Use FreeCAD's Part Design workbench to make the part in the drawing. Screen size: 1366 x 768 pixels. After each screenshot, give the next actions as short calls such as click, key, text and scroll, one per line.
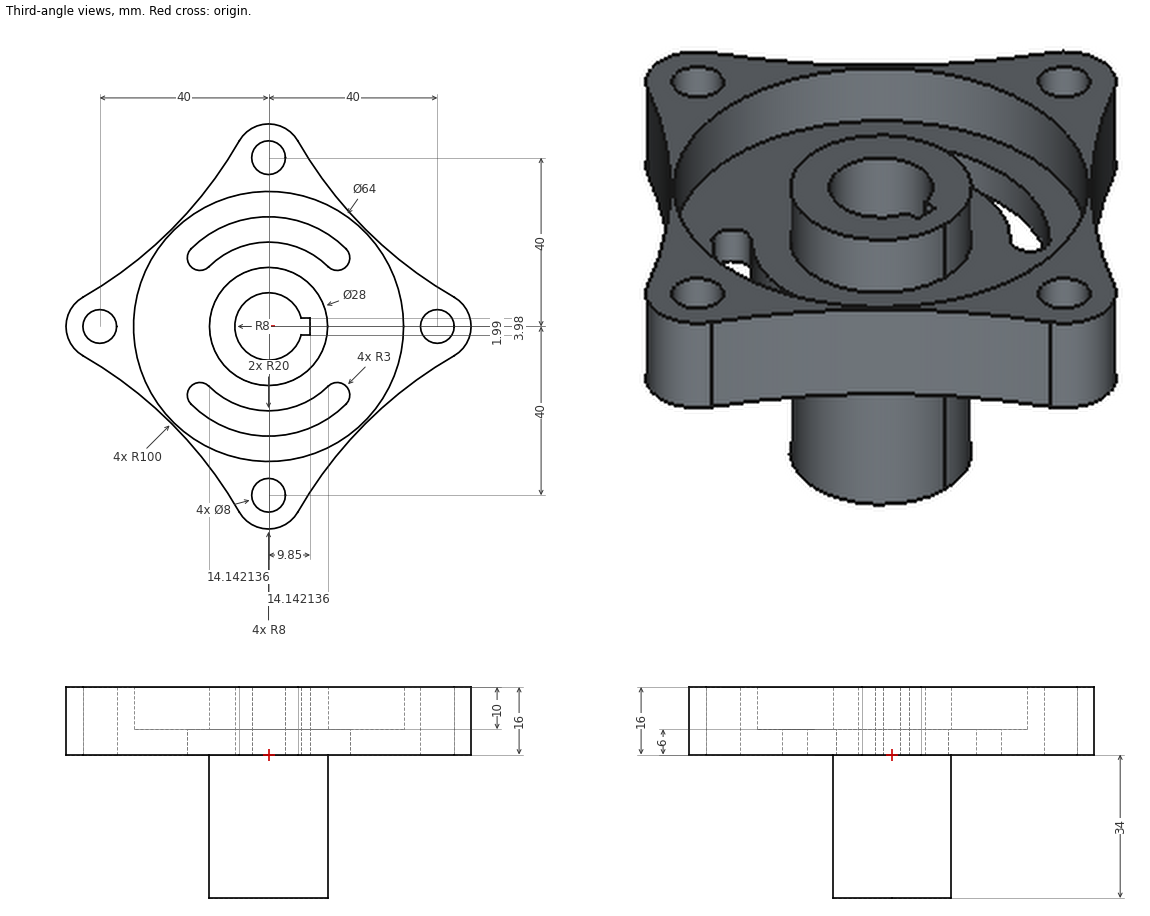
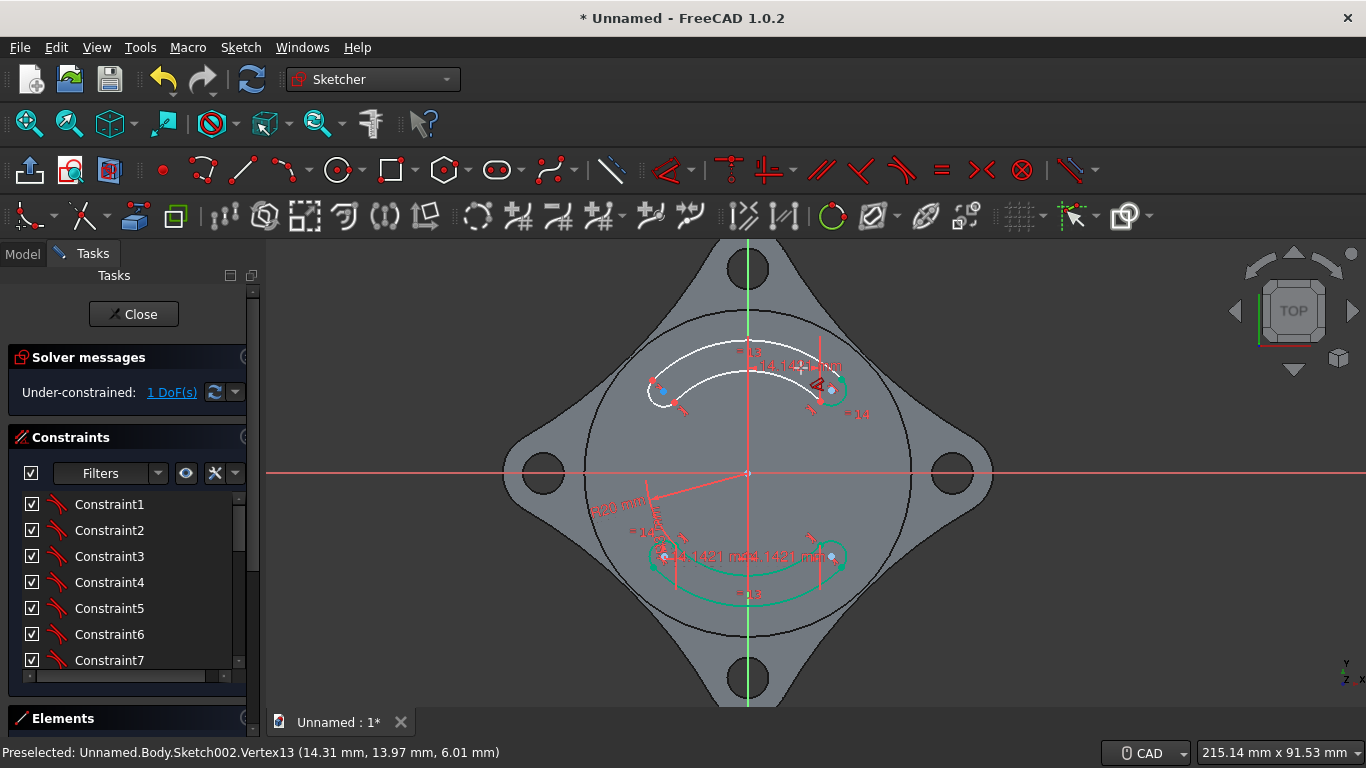
click(675, 402)
click(694, 368)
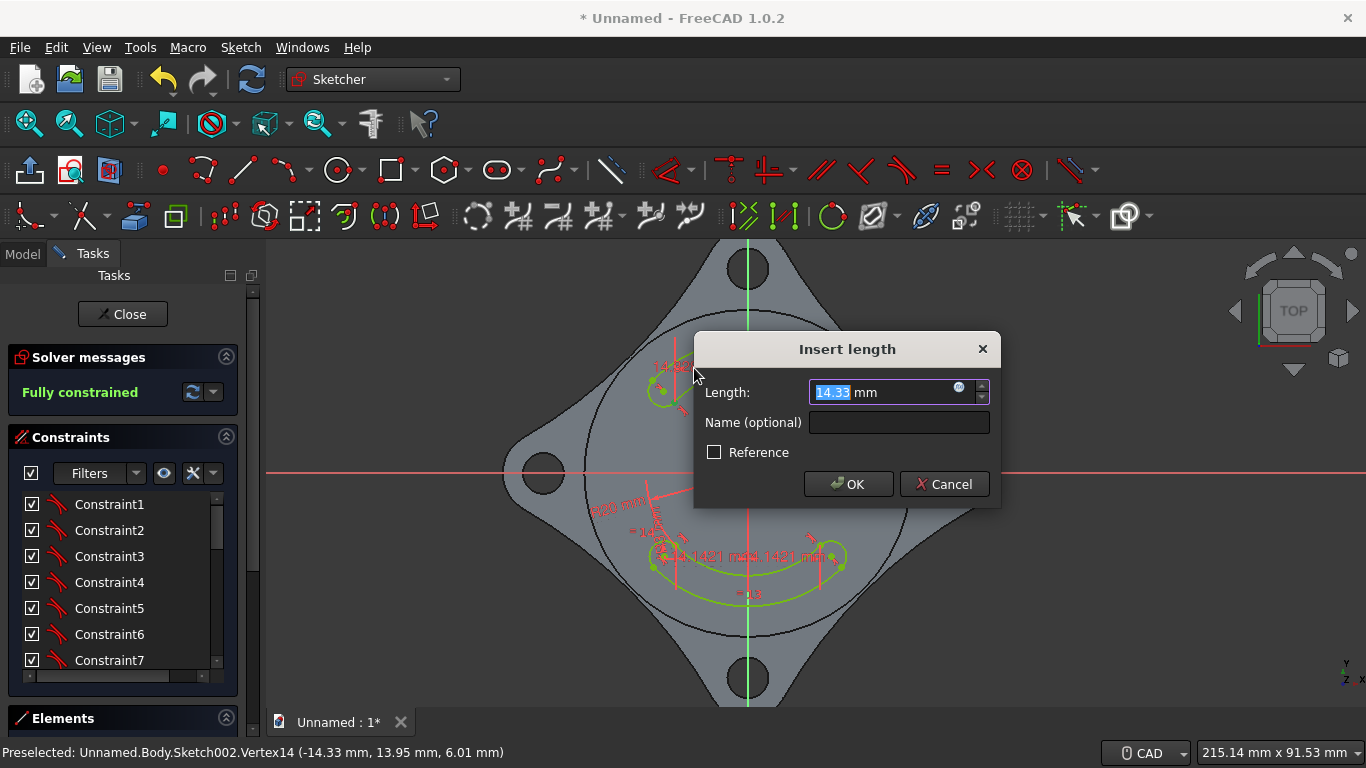
text(14.142136)
key(Return)
key(Escape)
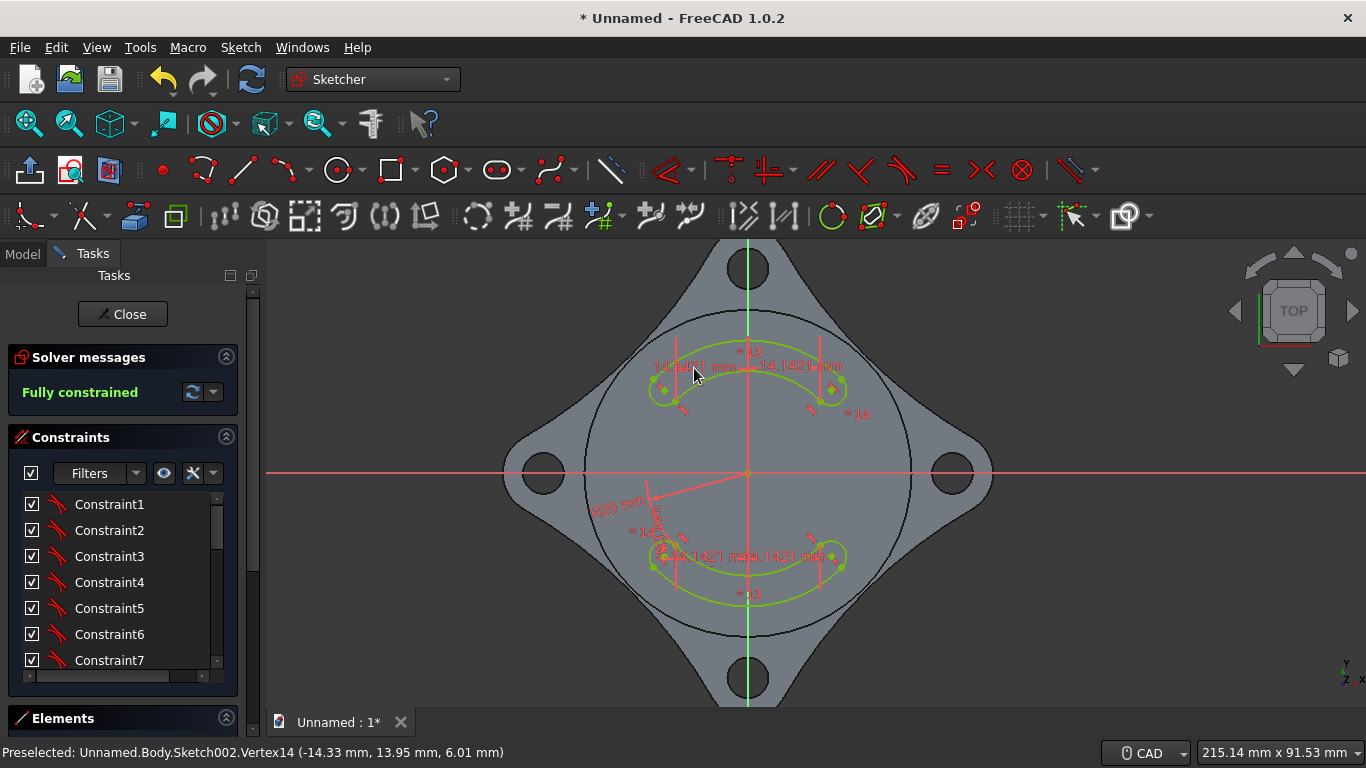
click(123, 314)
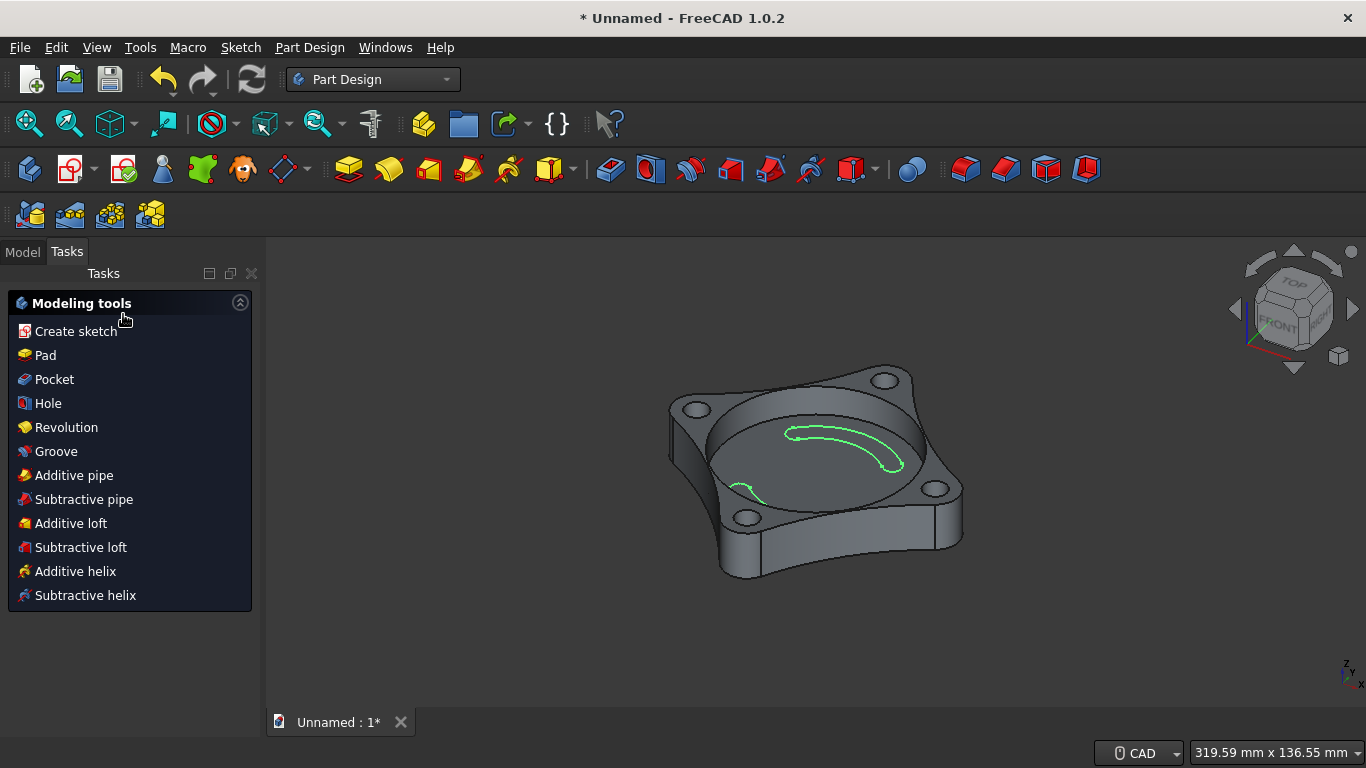
click(612, 170)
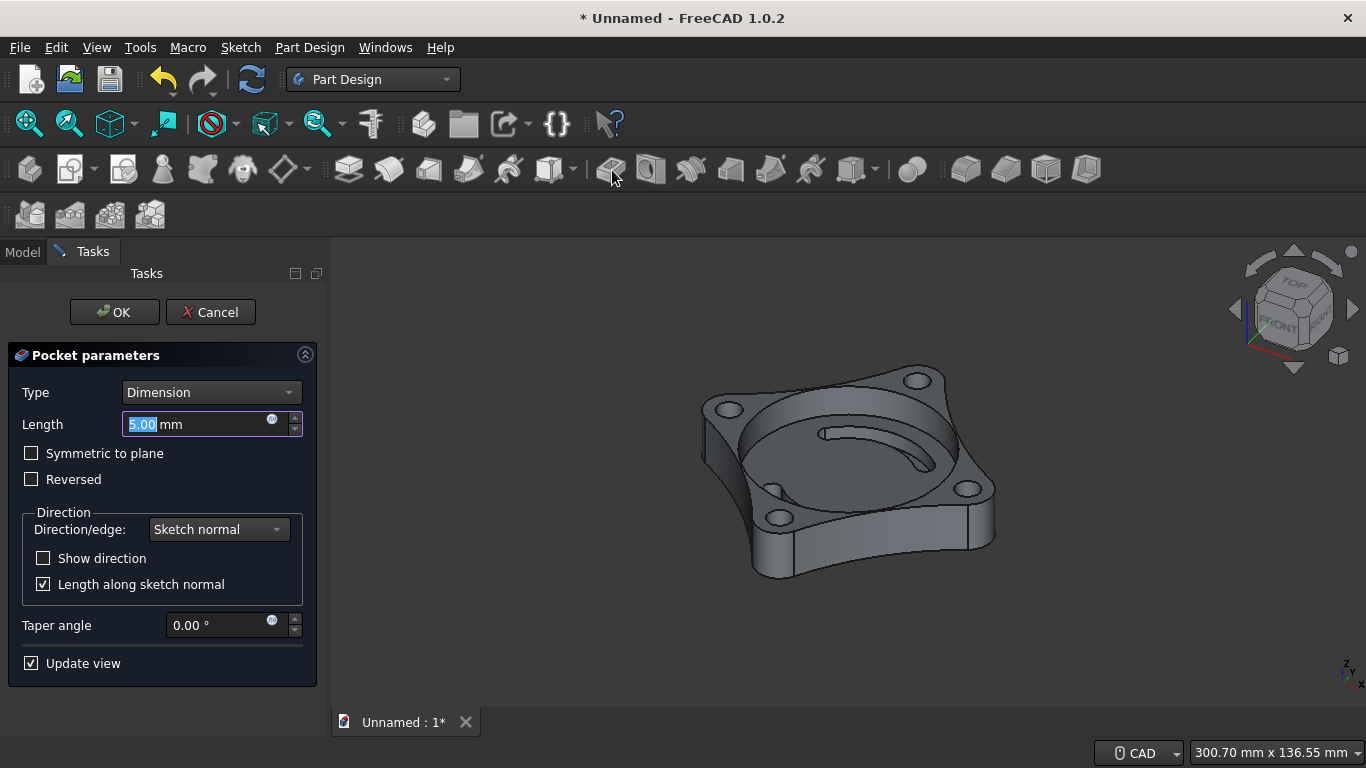
text(6)
key(Tab)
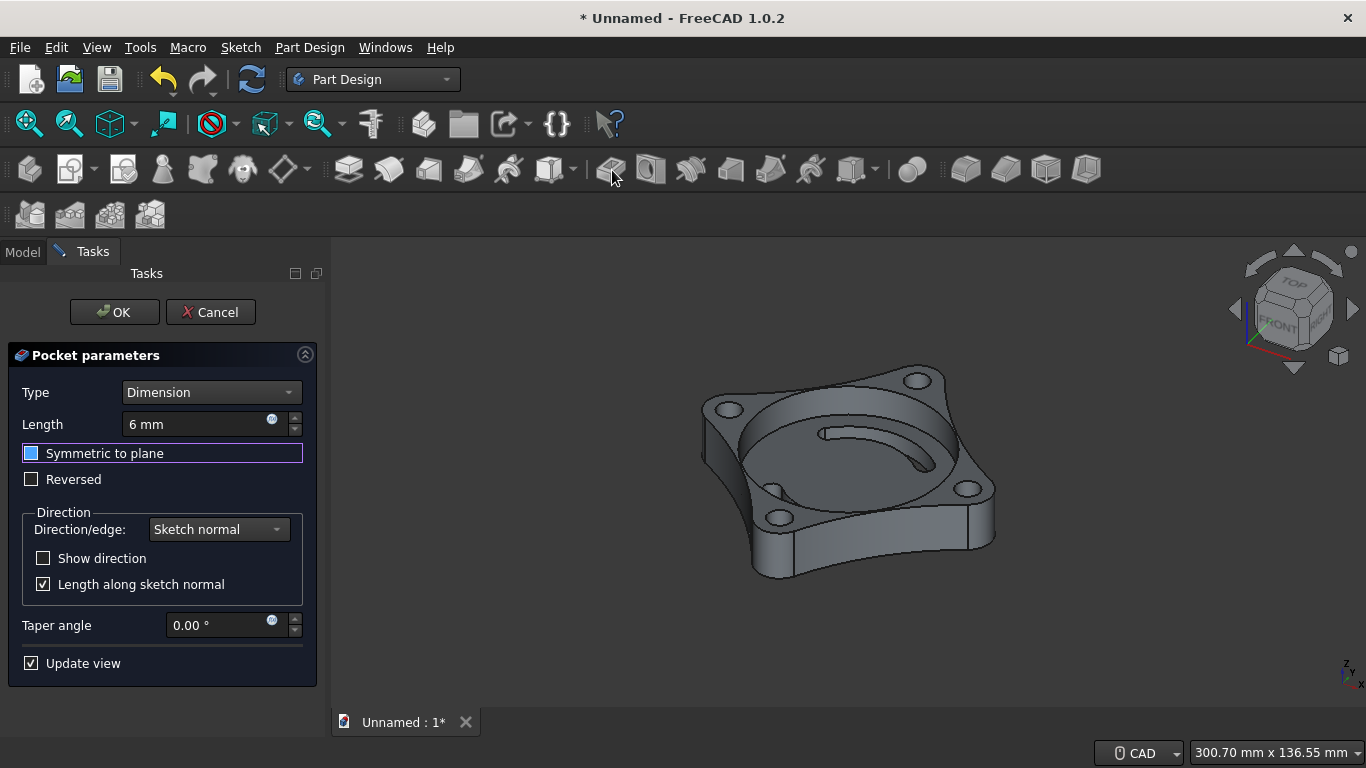
click(115, 312)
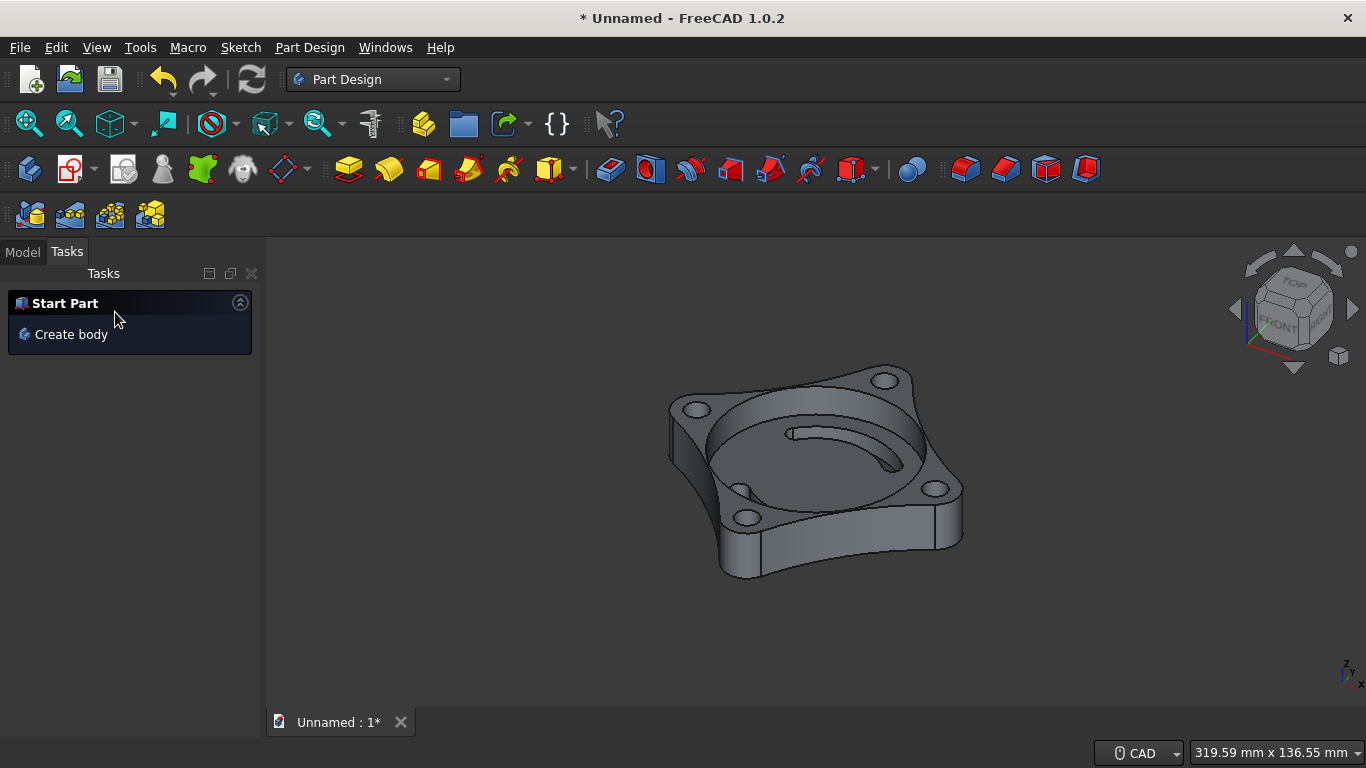
click(816, 477)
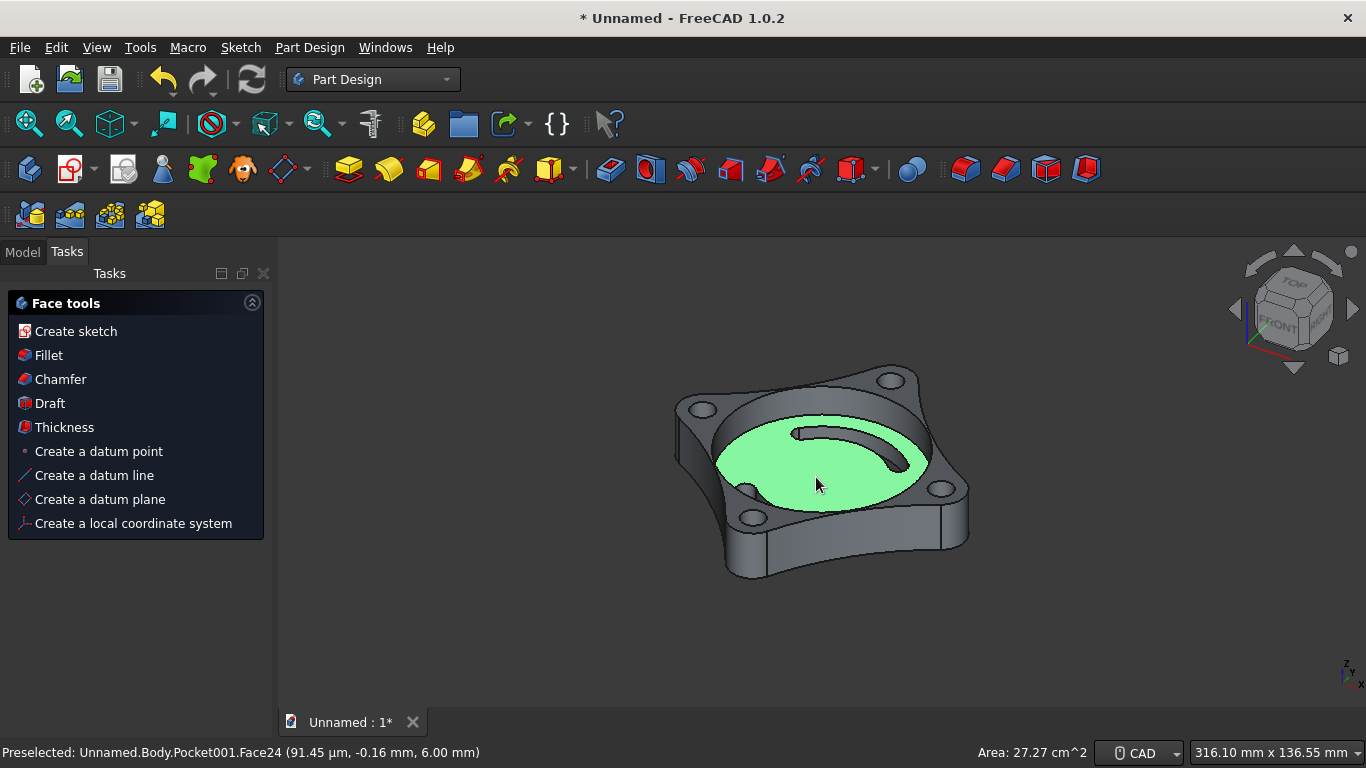
click(70, 170)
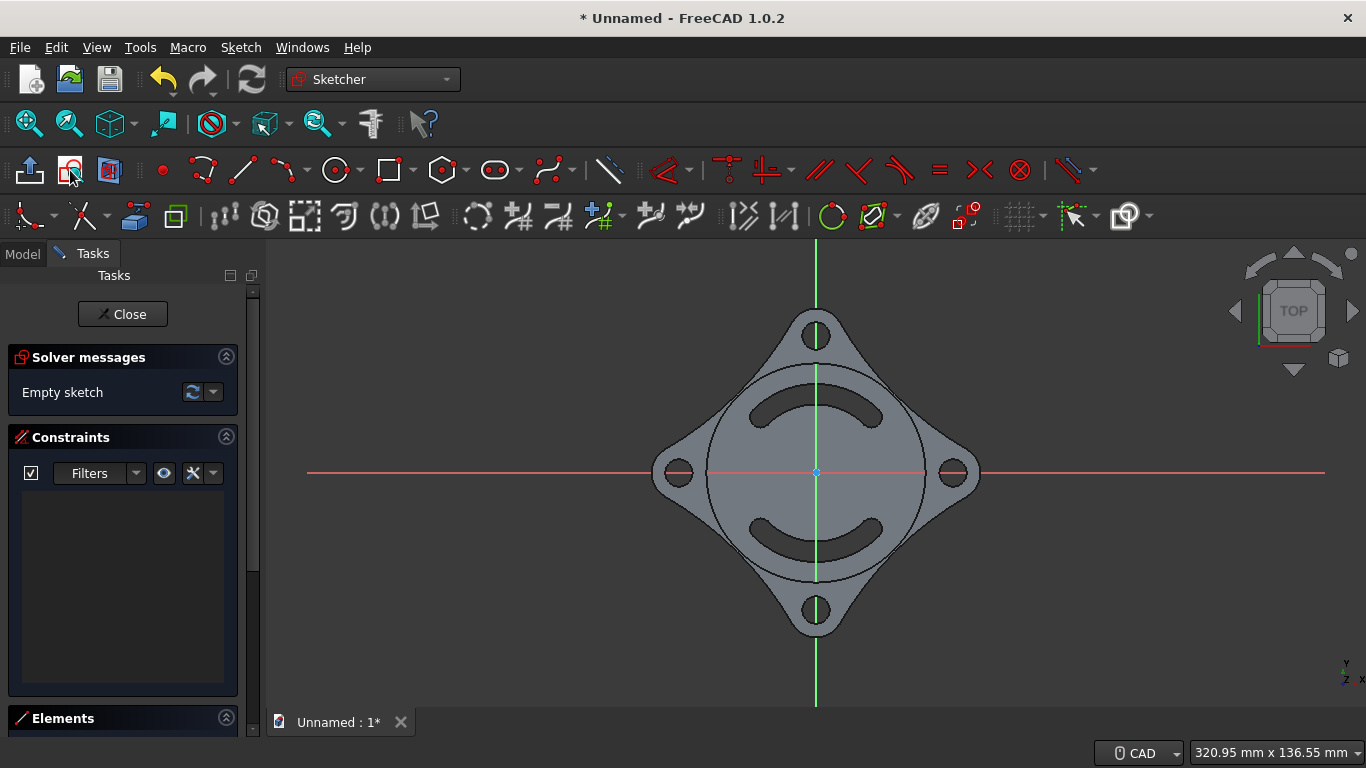
scroll(846, 473, up, 6)